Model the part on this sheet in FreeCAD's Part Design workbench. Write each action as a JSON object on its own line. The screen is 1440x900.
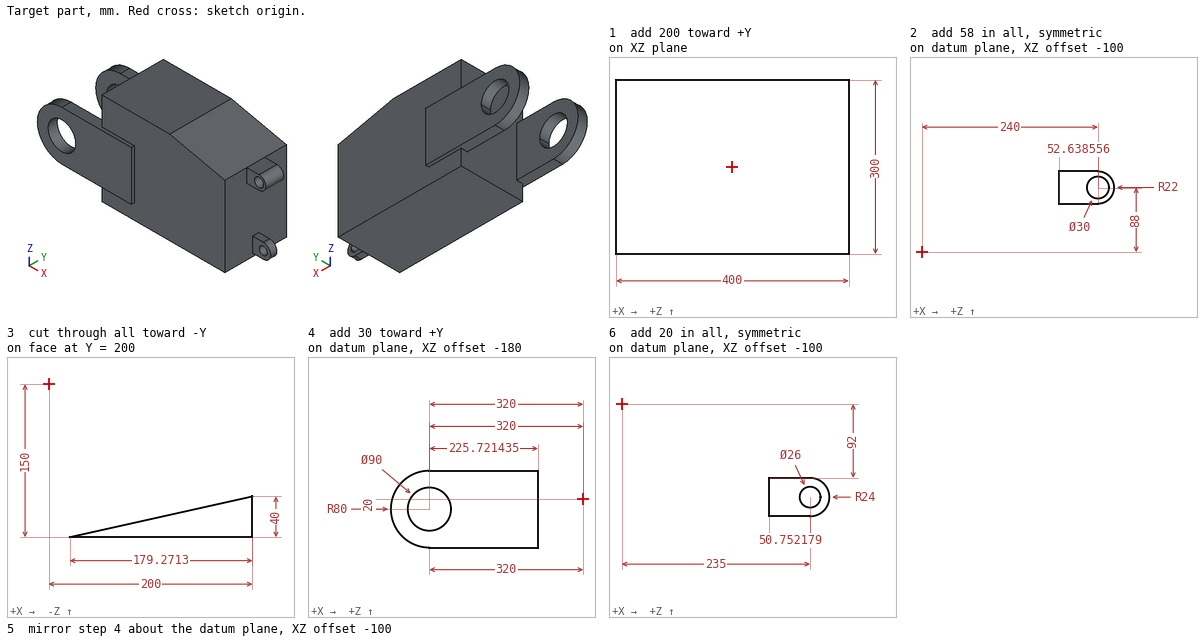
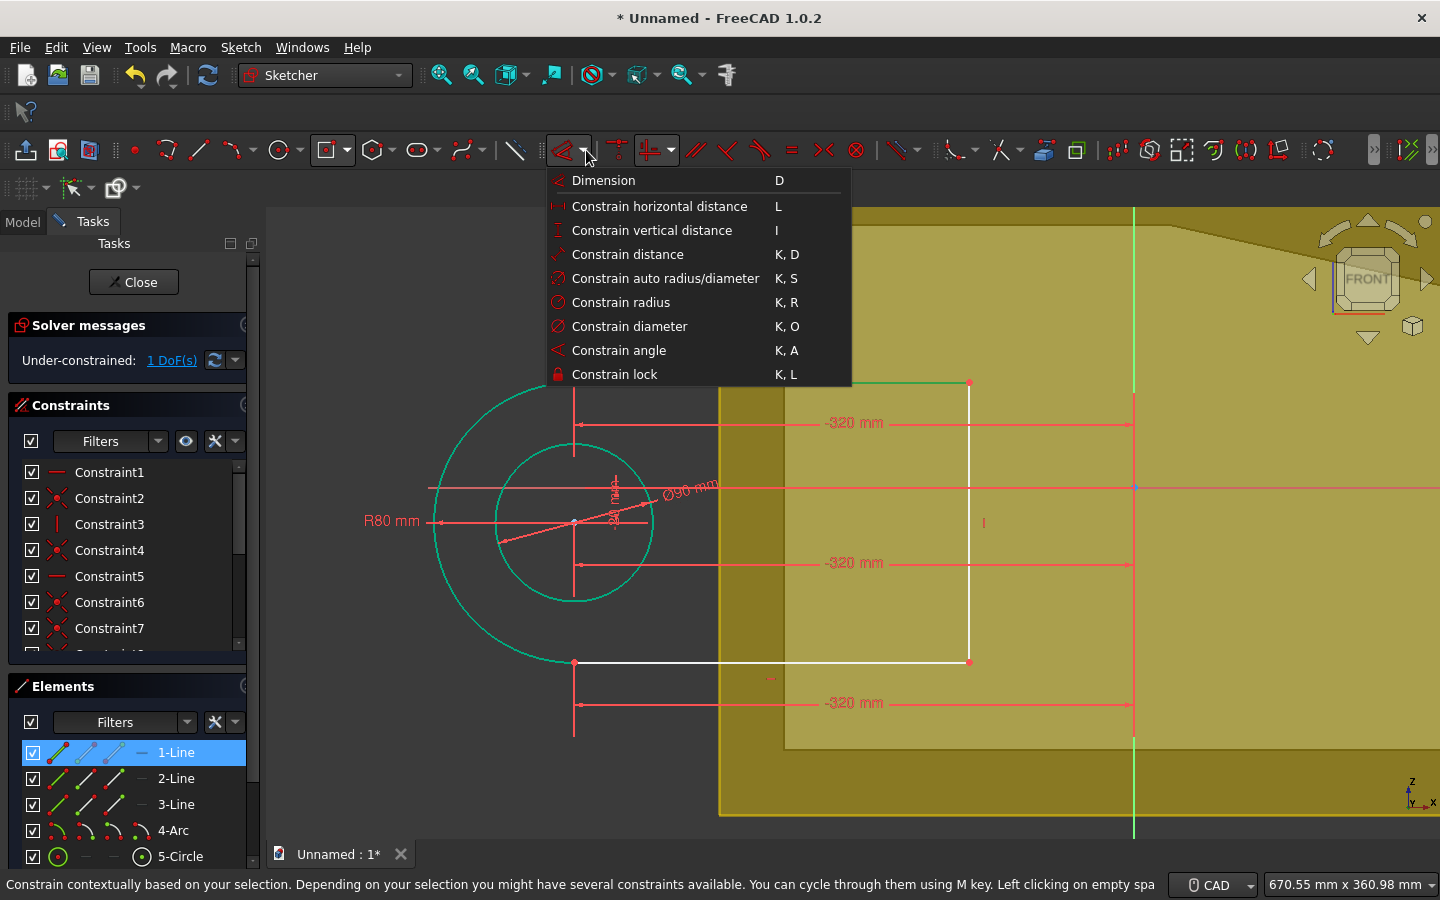
{"action": "left_click", "coordinate": [699, 206]}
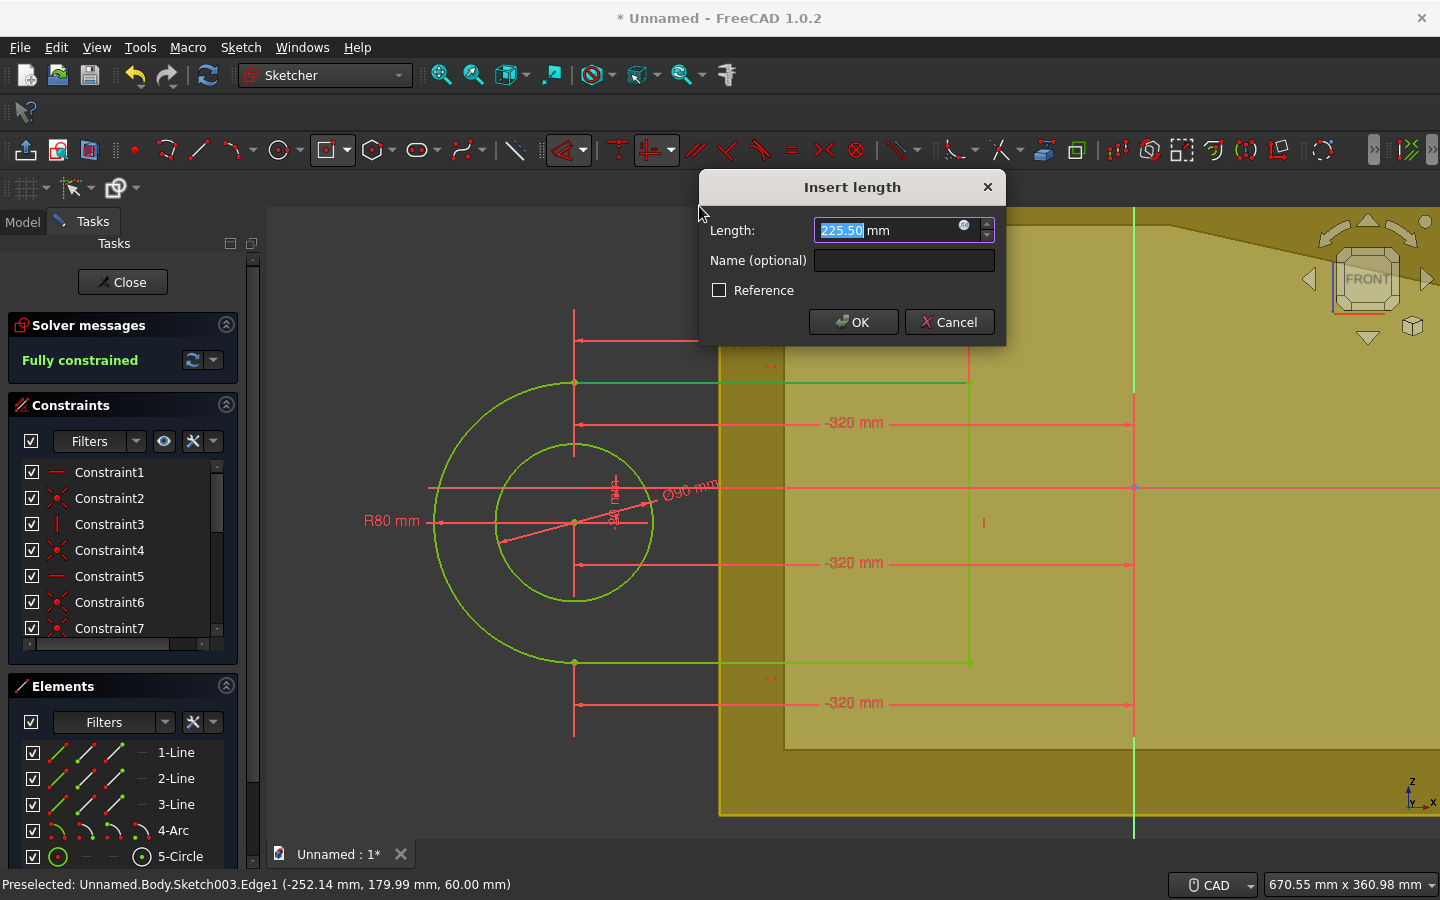
{"action": "type", "text": "225.721435"}
{"action": "key", "text": "Return"}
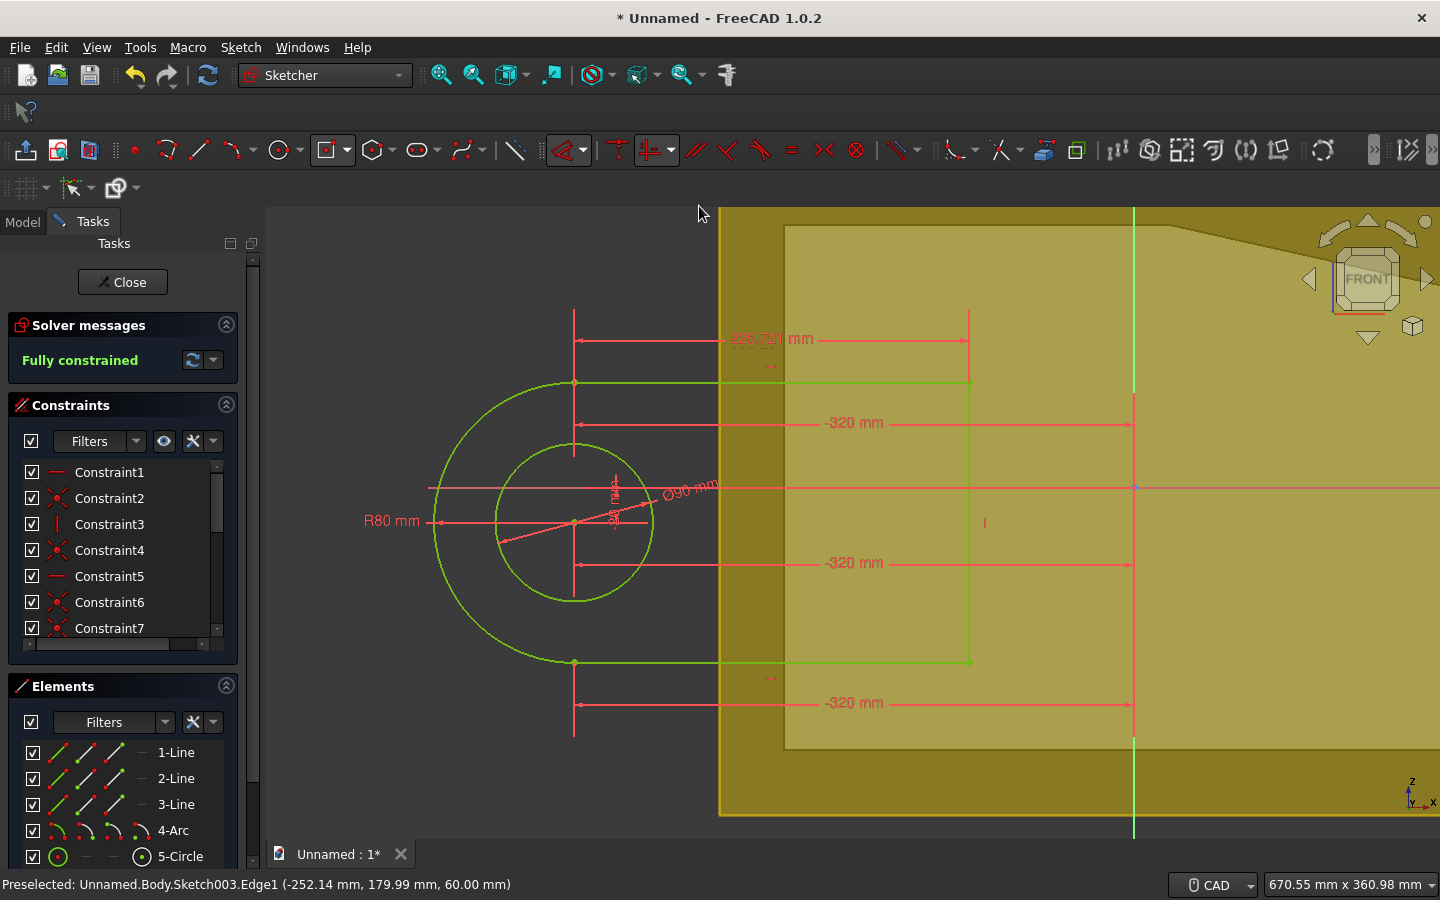
{"action": "left_click", "coordinate": [123, 282]}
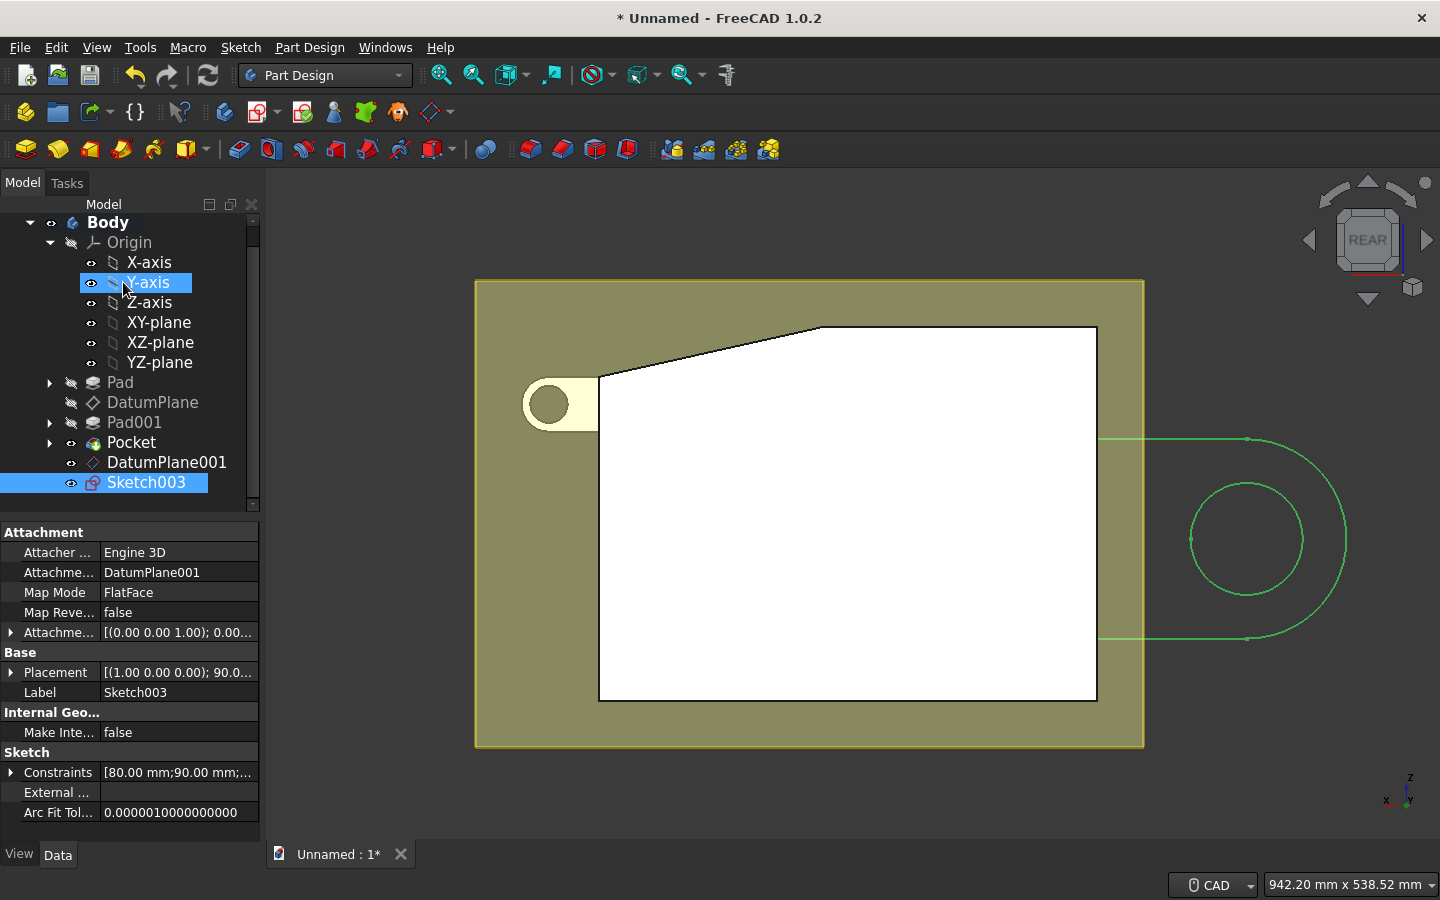
{"action": "left_click", "coordinate": [26, 150]}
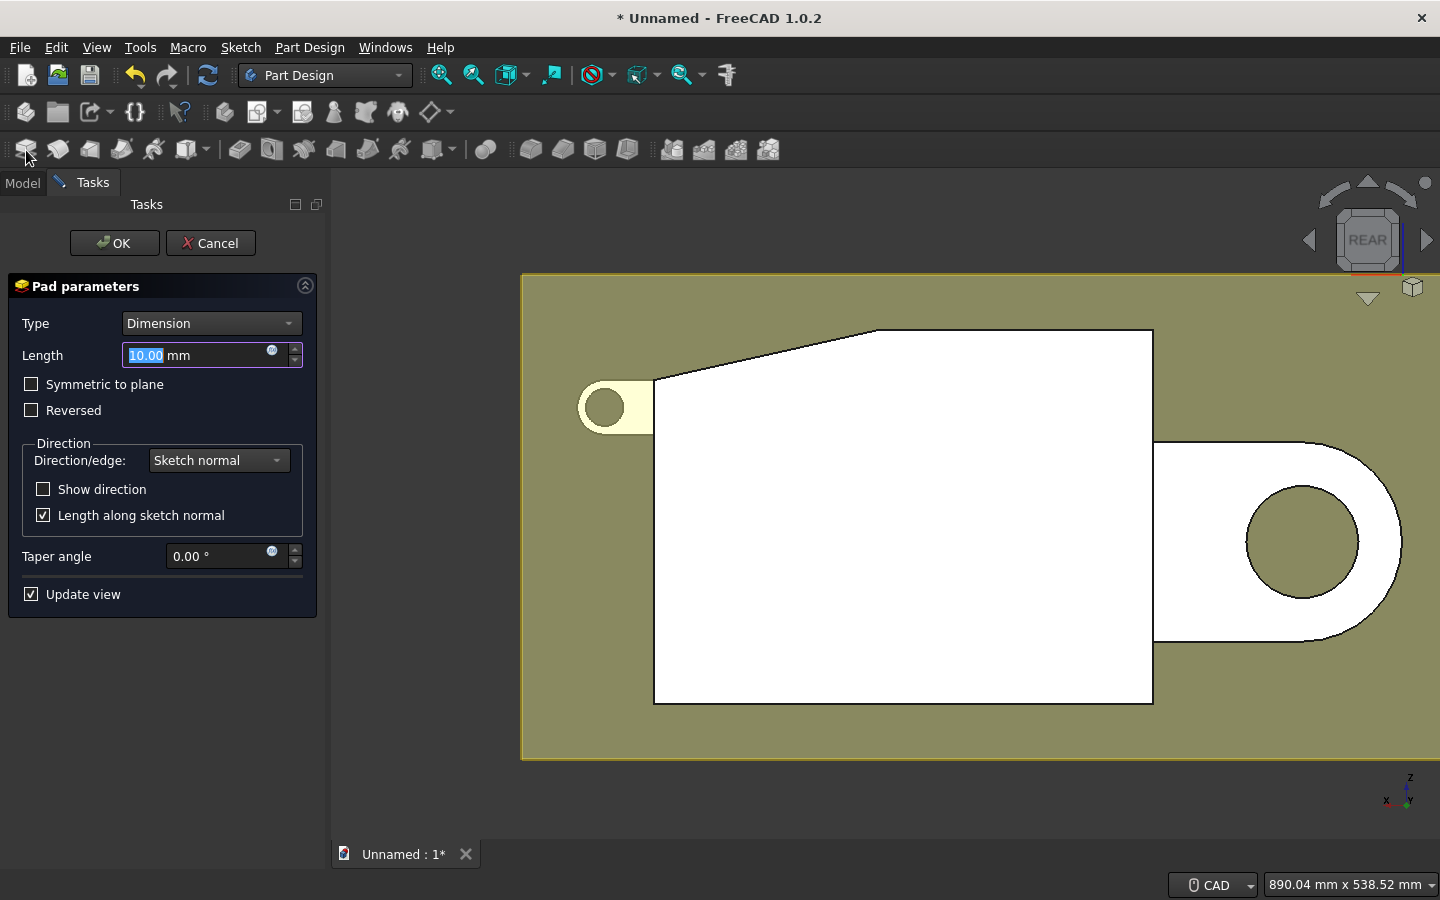
{"action": "type", "text": "30"}
{"action": "key", "text": "Tab"}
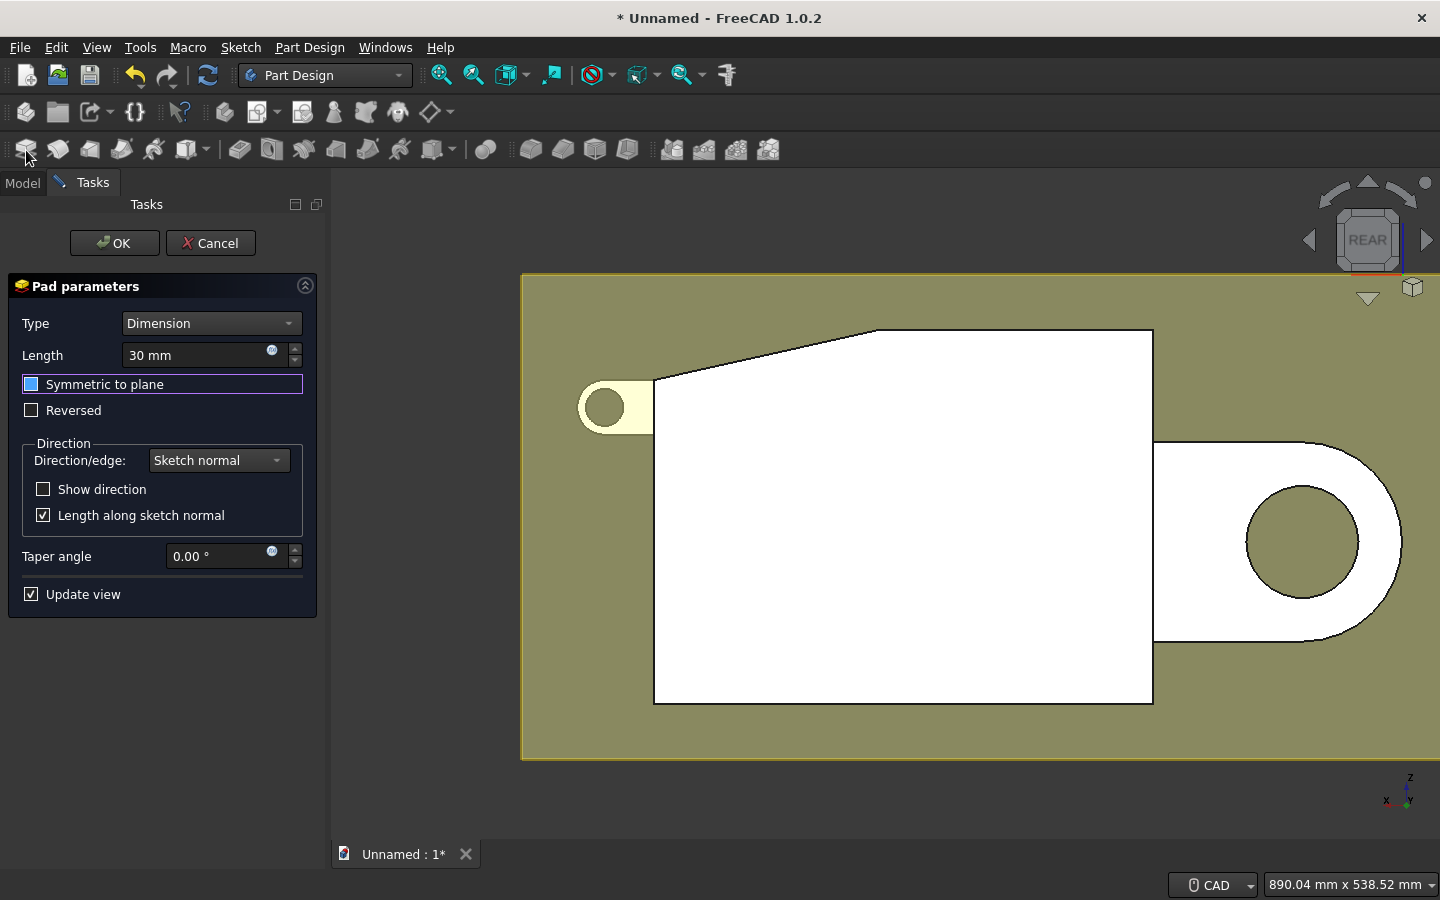
{"action": "left_click", "coordinate": [30, 410]}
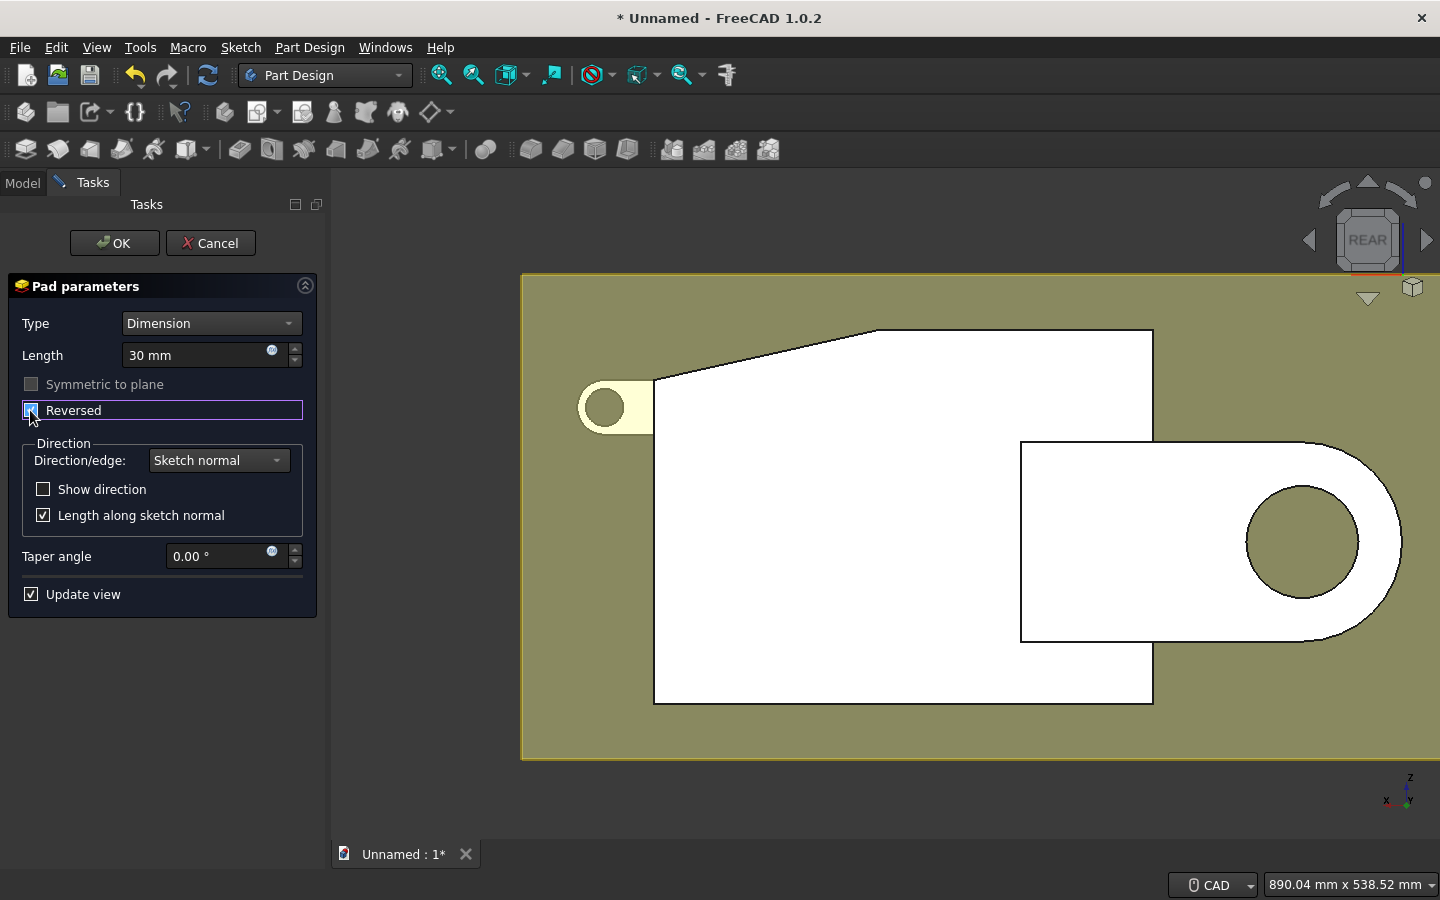
{"action": "left_click", "coordinate": [115, 243]}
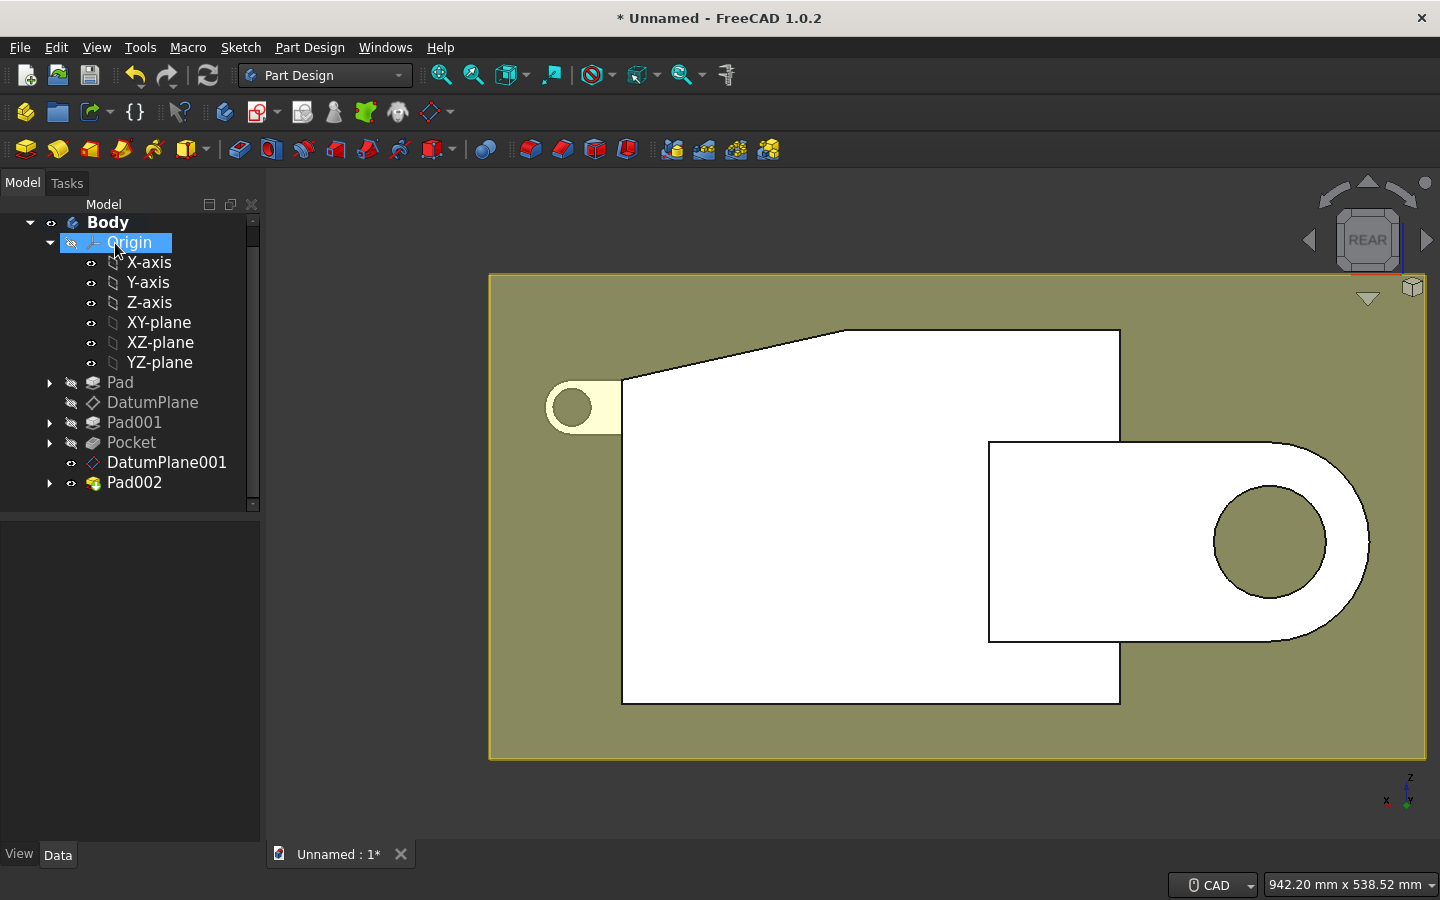
{"action": "left_click", "coordinate": [116, 463]}
{"action": "key", "text": "space"}